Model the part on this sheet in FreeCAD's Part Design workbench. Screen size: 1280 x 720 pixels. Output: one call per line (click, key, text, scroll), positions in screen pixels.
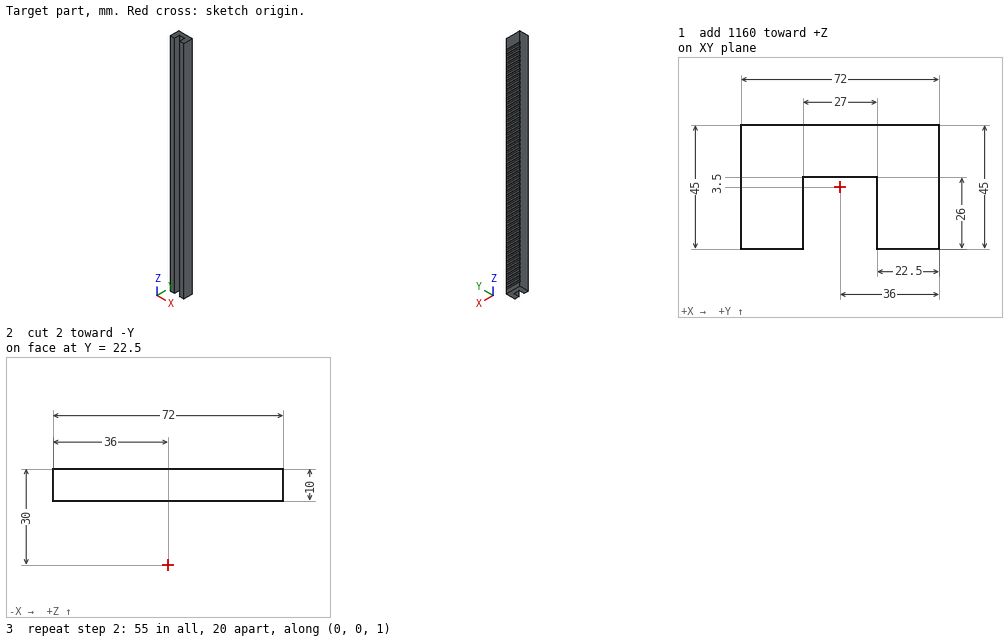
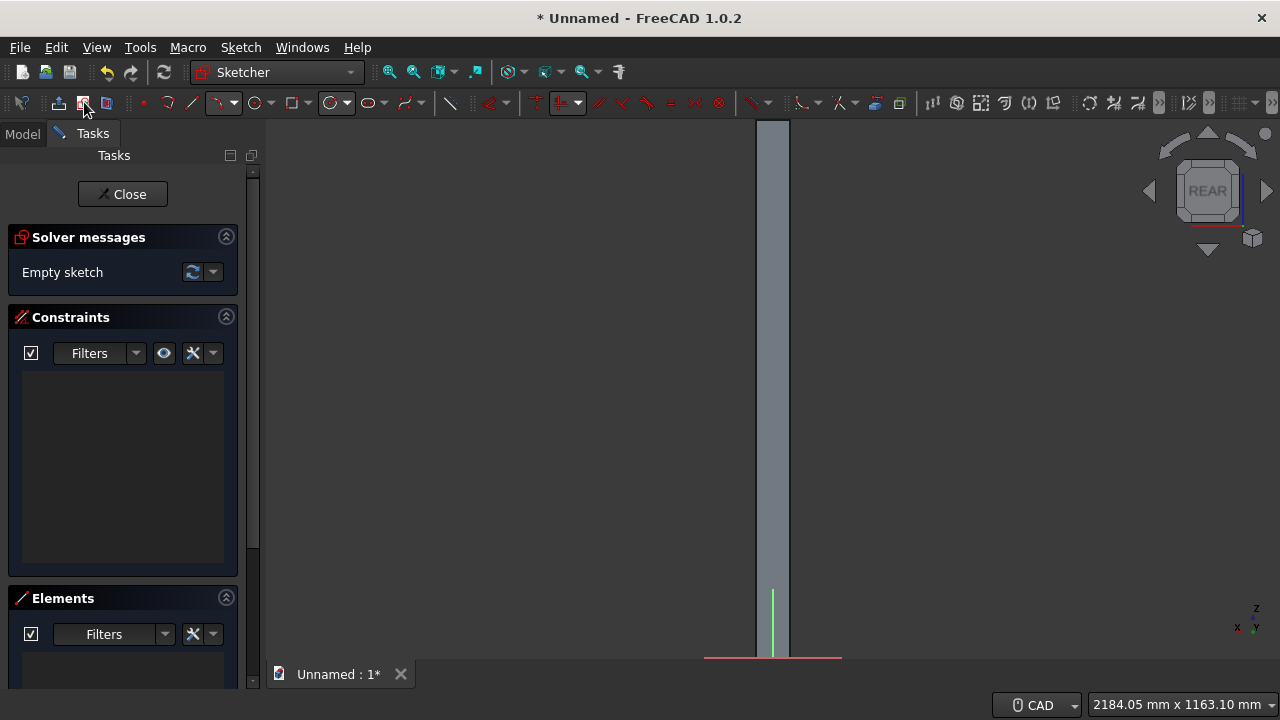
scroll(704, 389, down, 5)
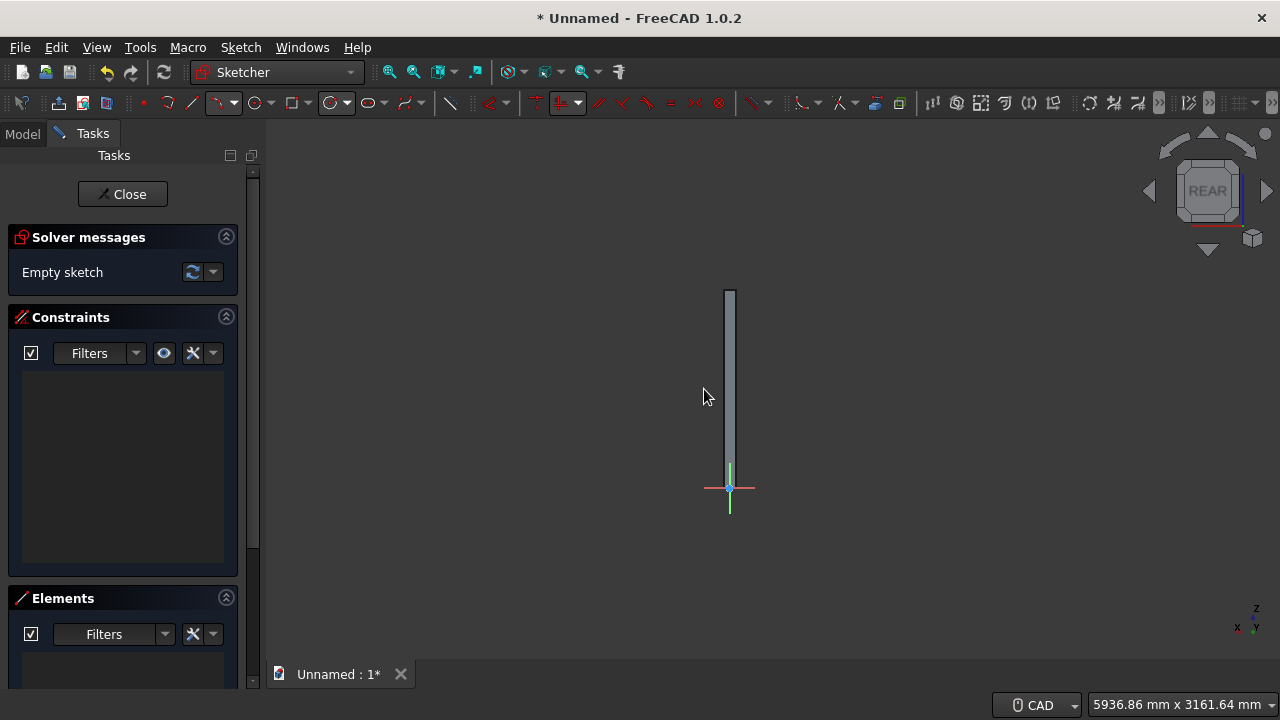
scroll(731, 491, up, 15)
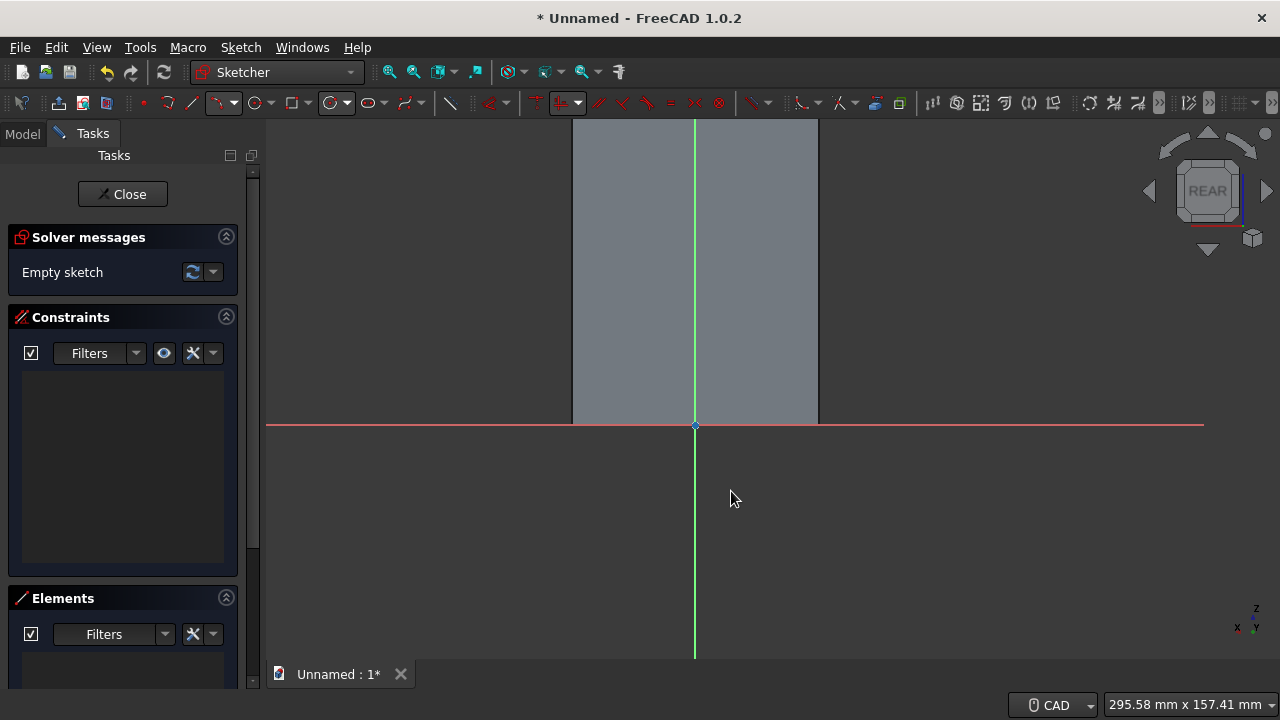
scroll(688, 361, up, 4)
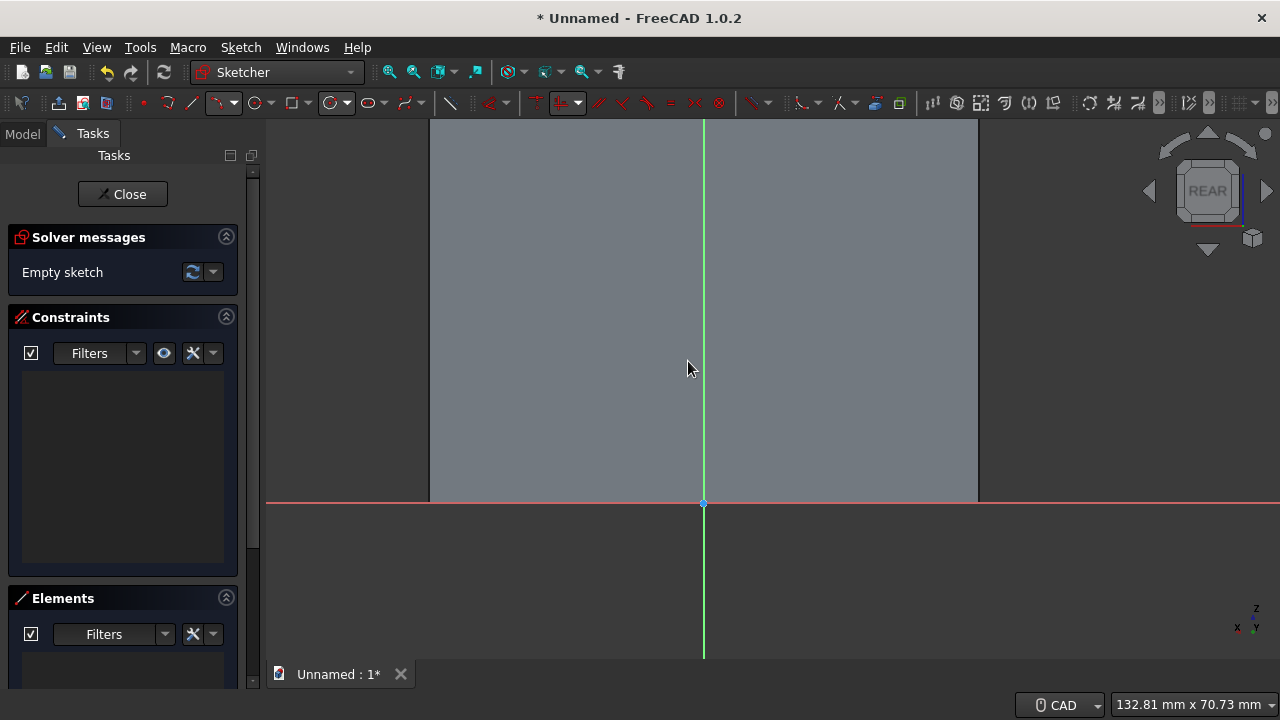
click(292, 104)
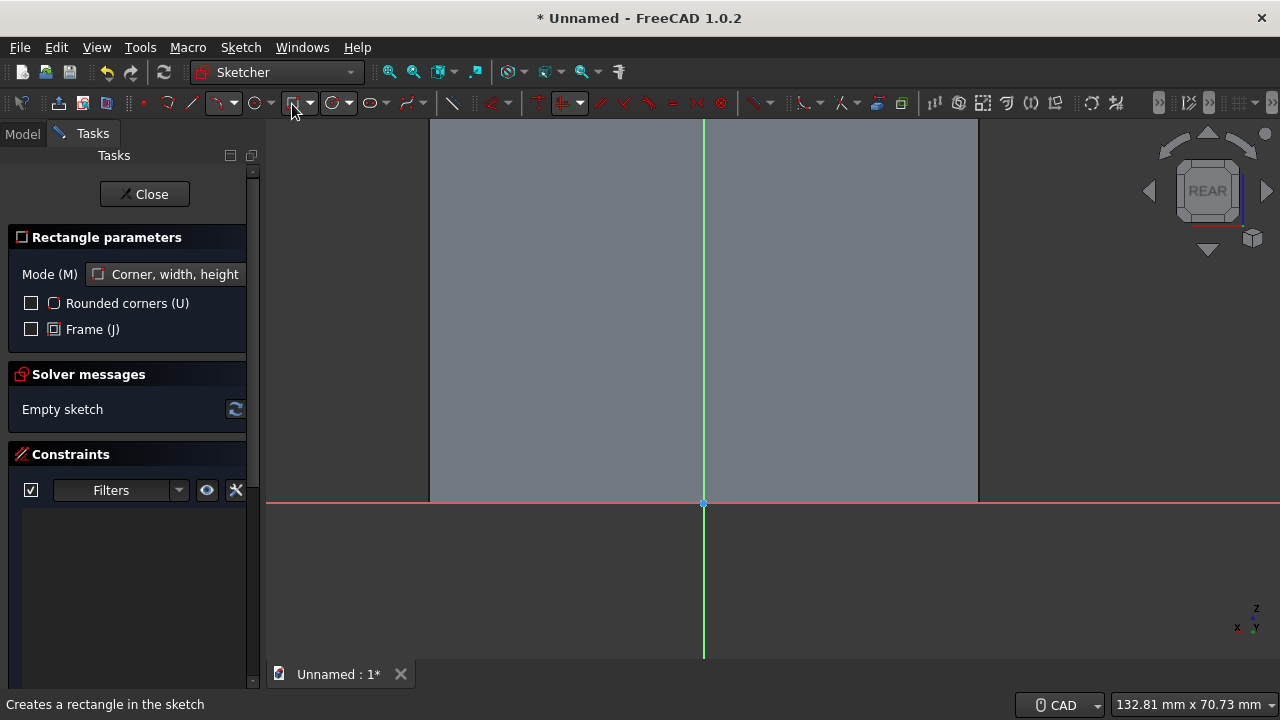
click(429, 274)
move(979, 351)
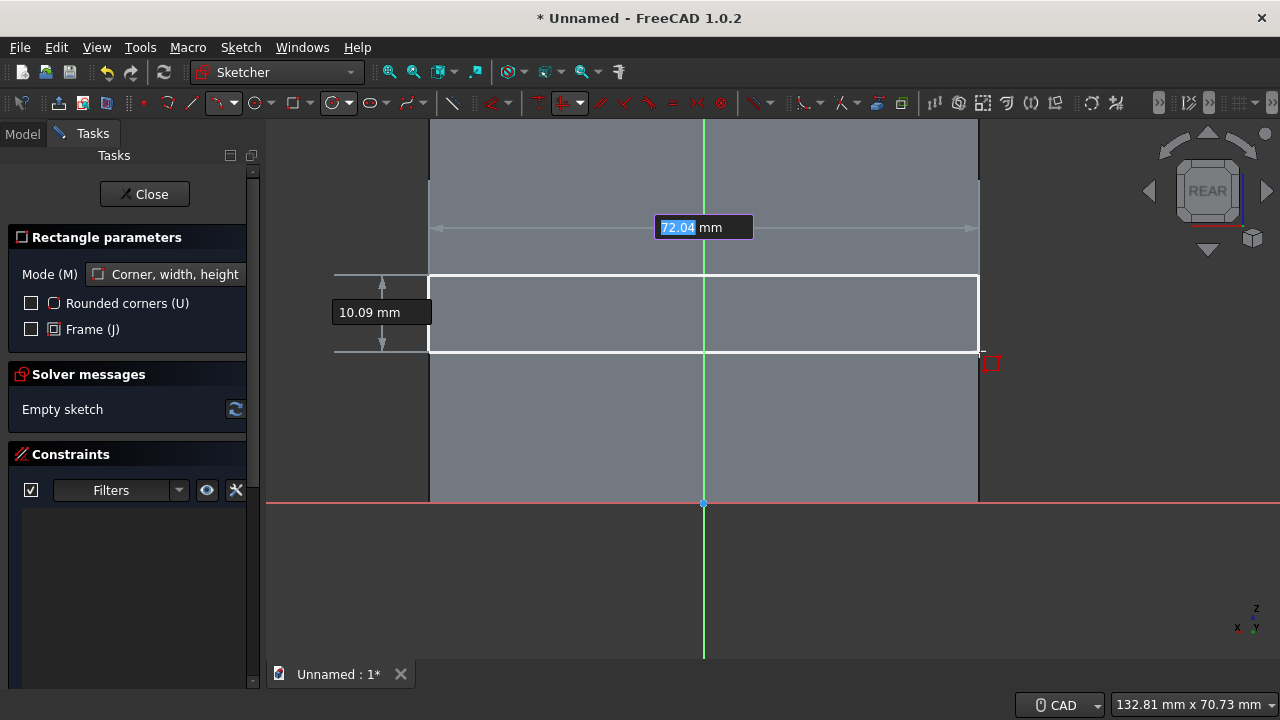
text(72)
key(Tab)
text(10)
key(Return)
key(Escape)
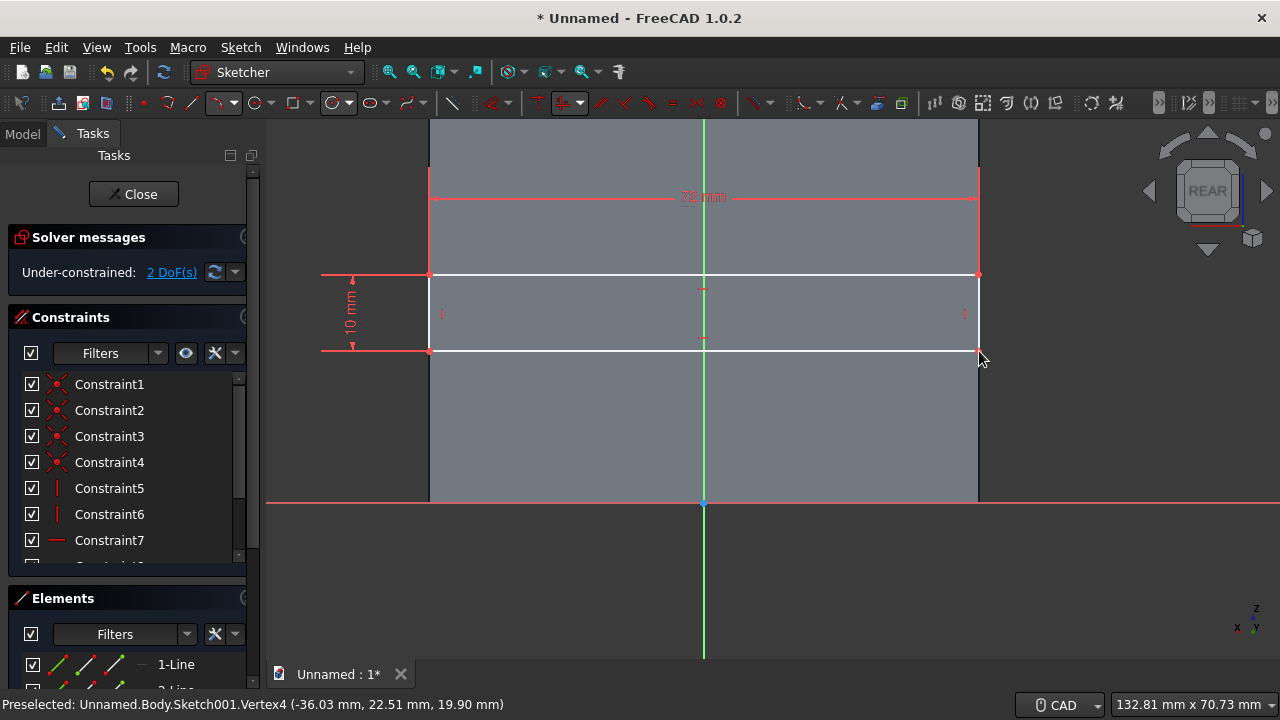
key(d)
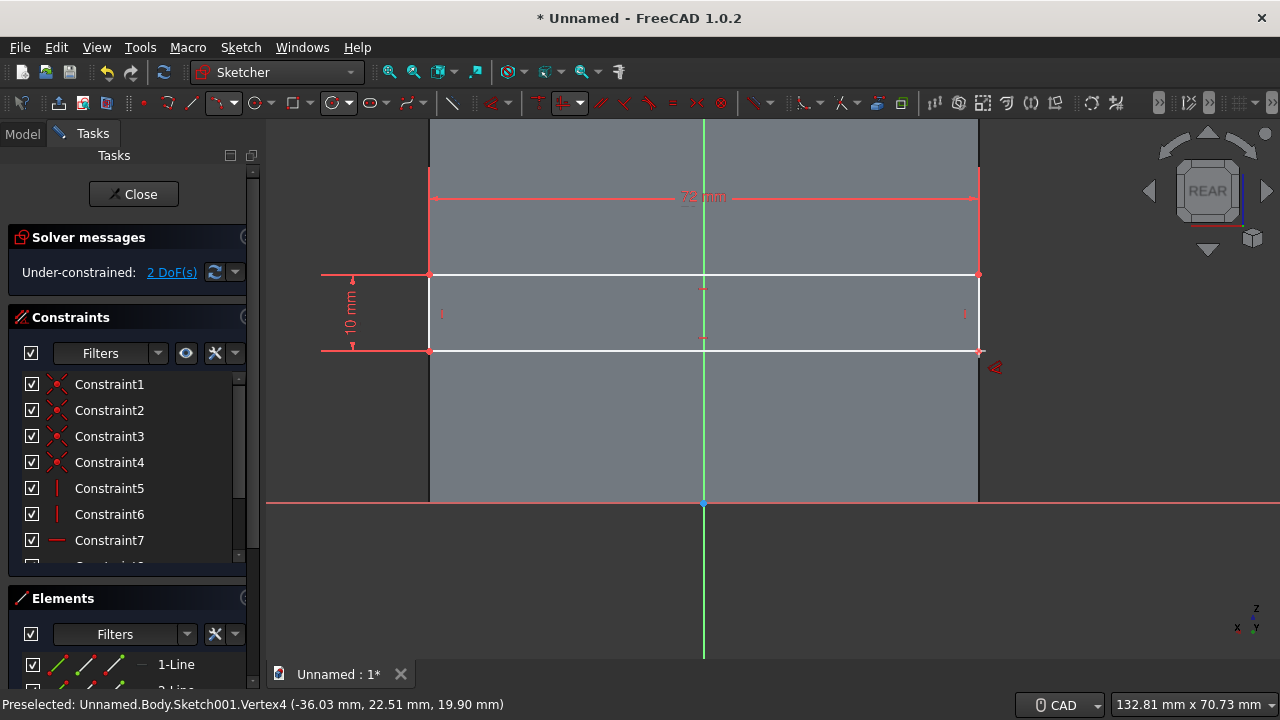
click(429, 275)
click(566, 537)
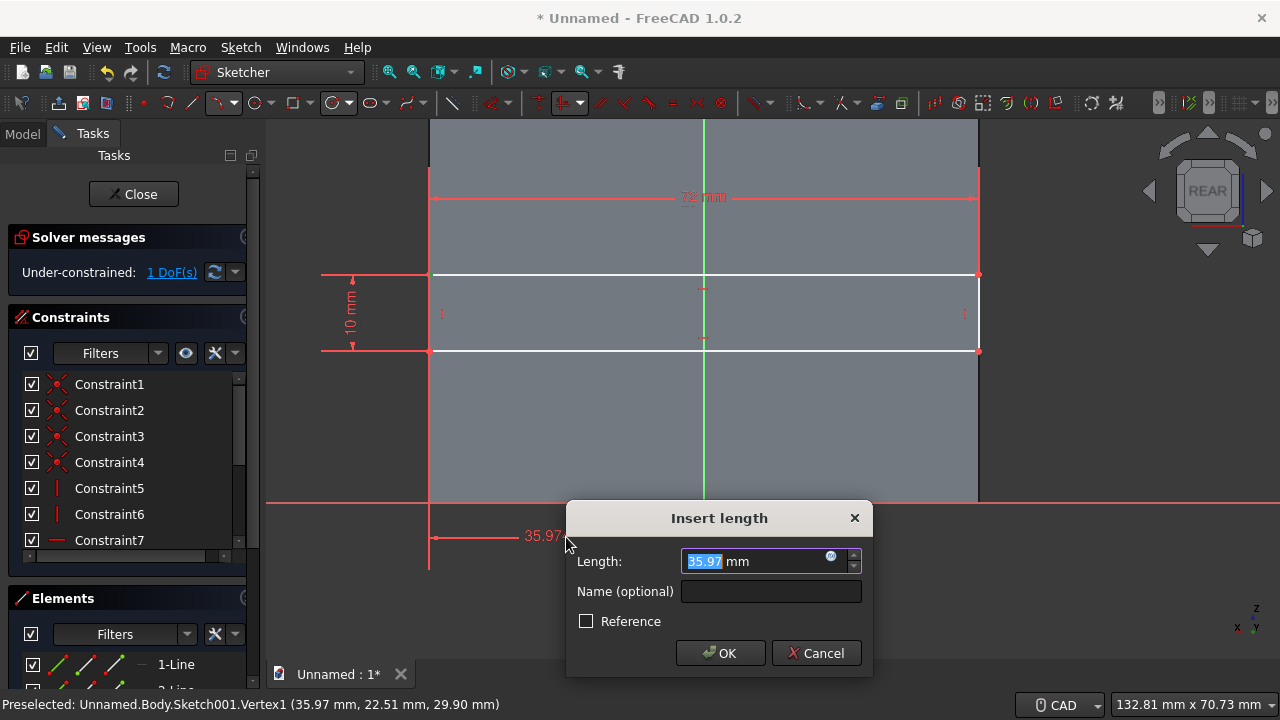
text(36)
key(Return)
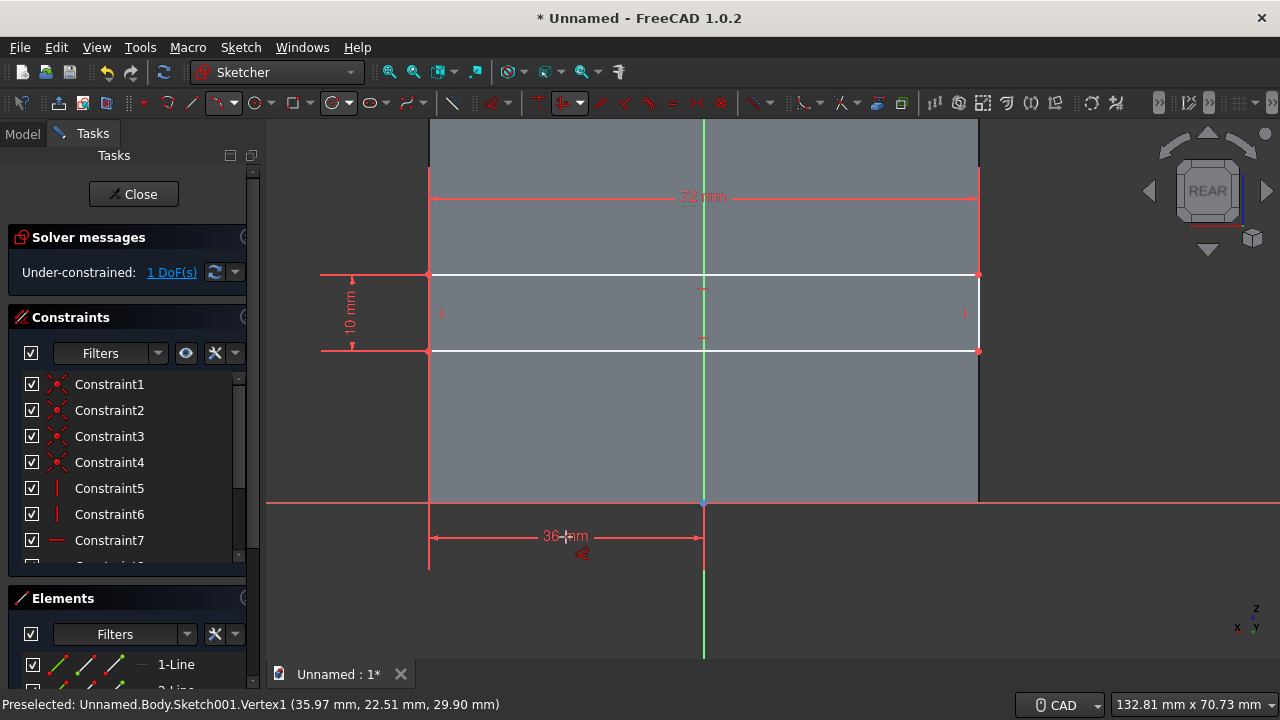
click(429, 275)
click(395, 389)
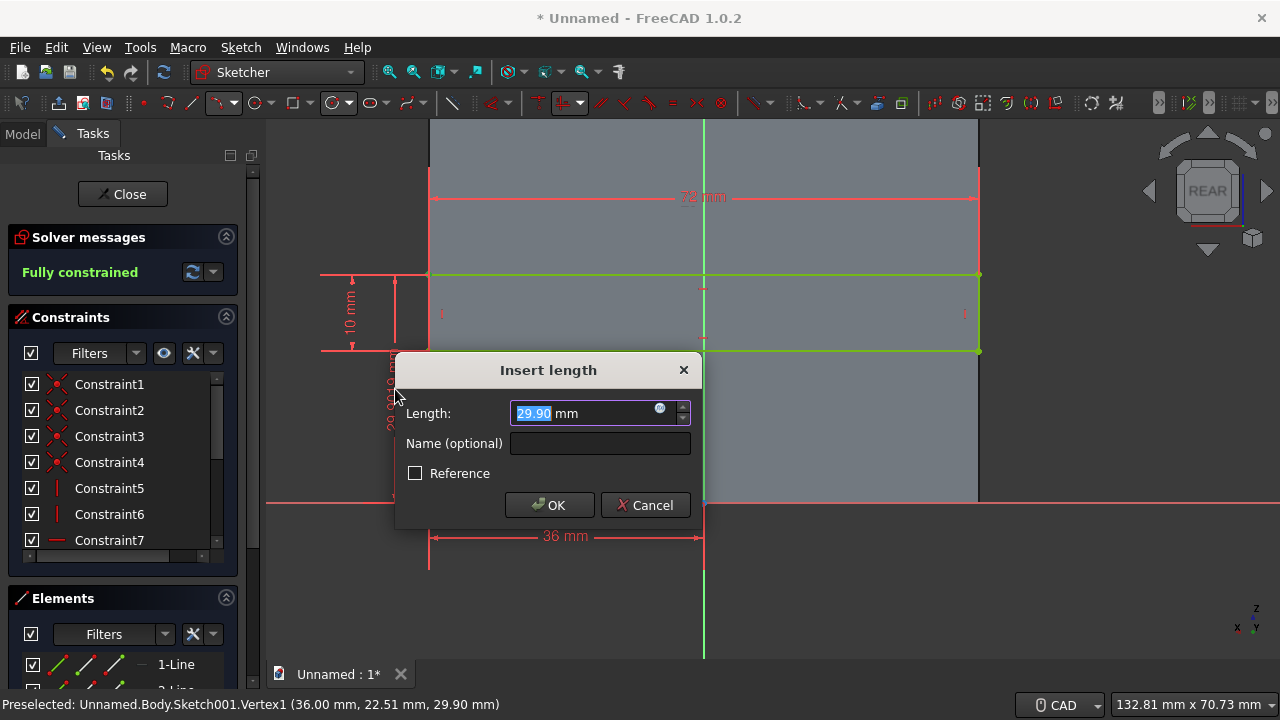
text(30)
key(Return)
key(Escape)